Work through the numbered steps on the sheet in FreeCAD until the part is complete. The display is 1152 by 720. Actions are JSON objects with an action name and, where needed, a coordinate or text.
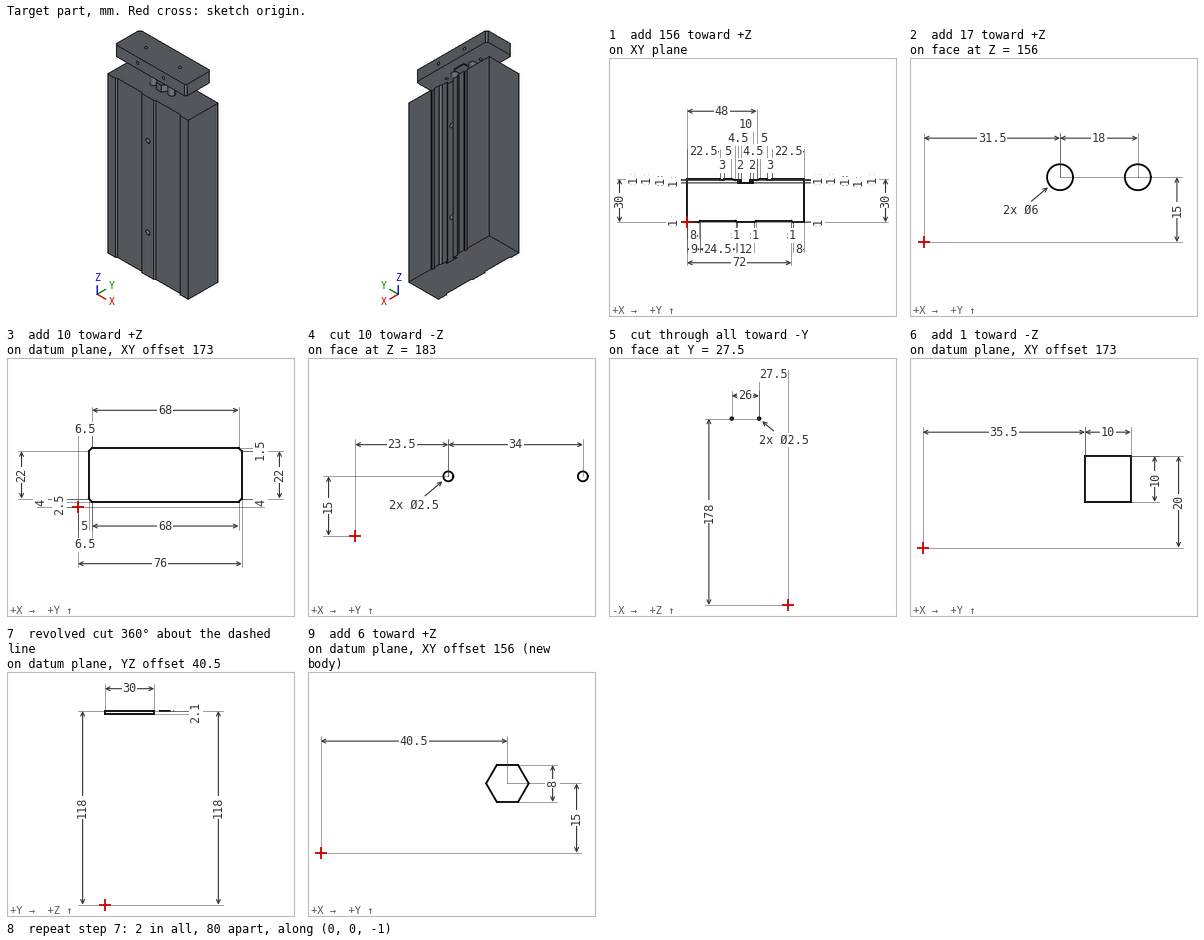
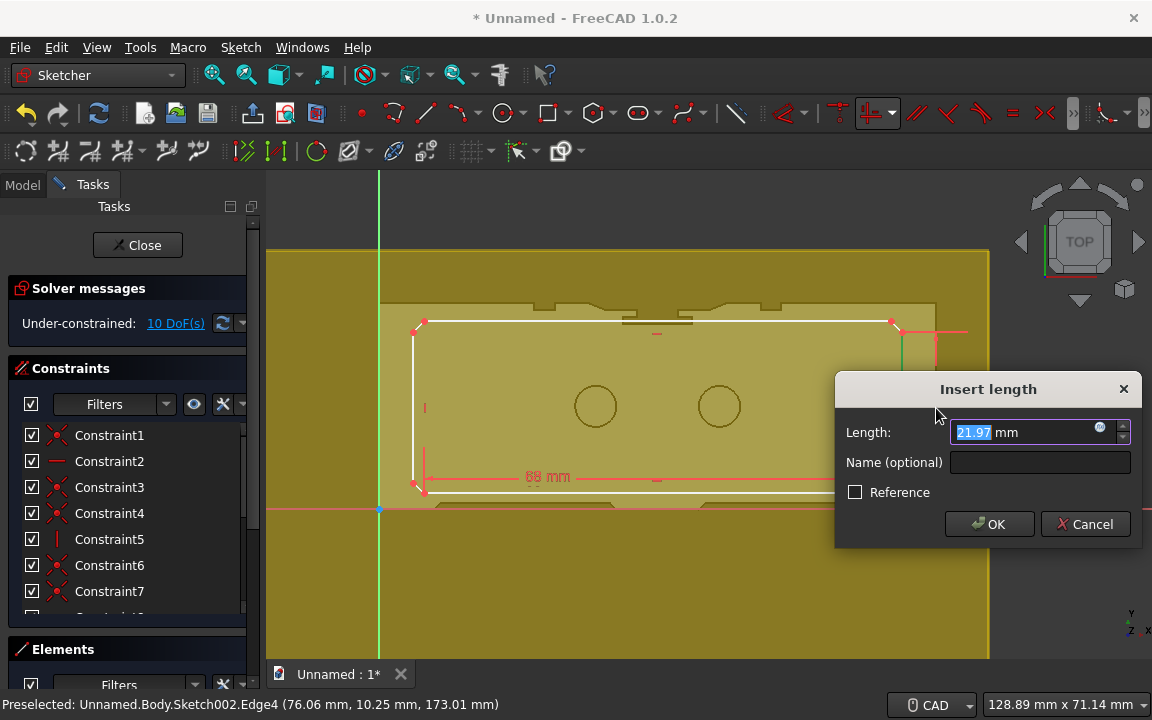
{"action": "type", "text": "22"}
{"action": "key", "text": "Return"}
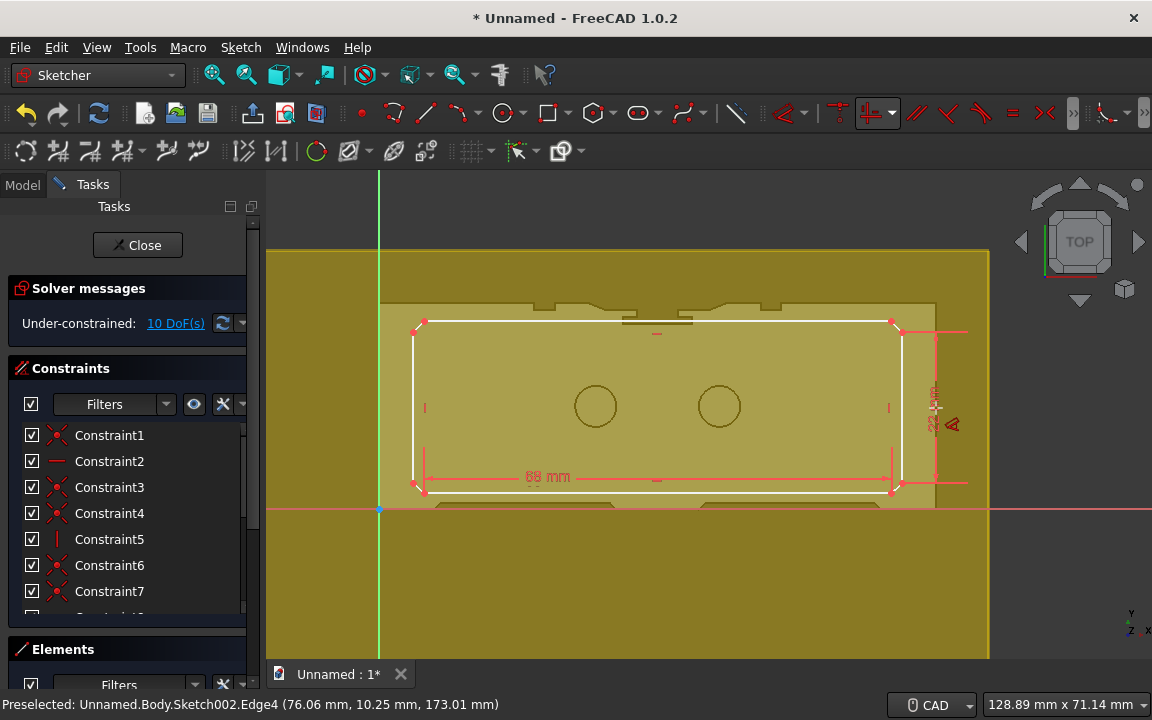
{"action": "left_click", "coordinate": [751, 321]}
{"action": "left_click", "coordinate": [658, 287]}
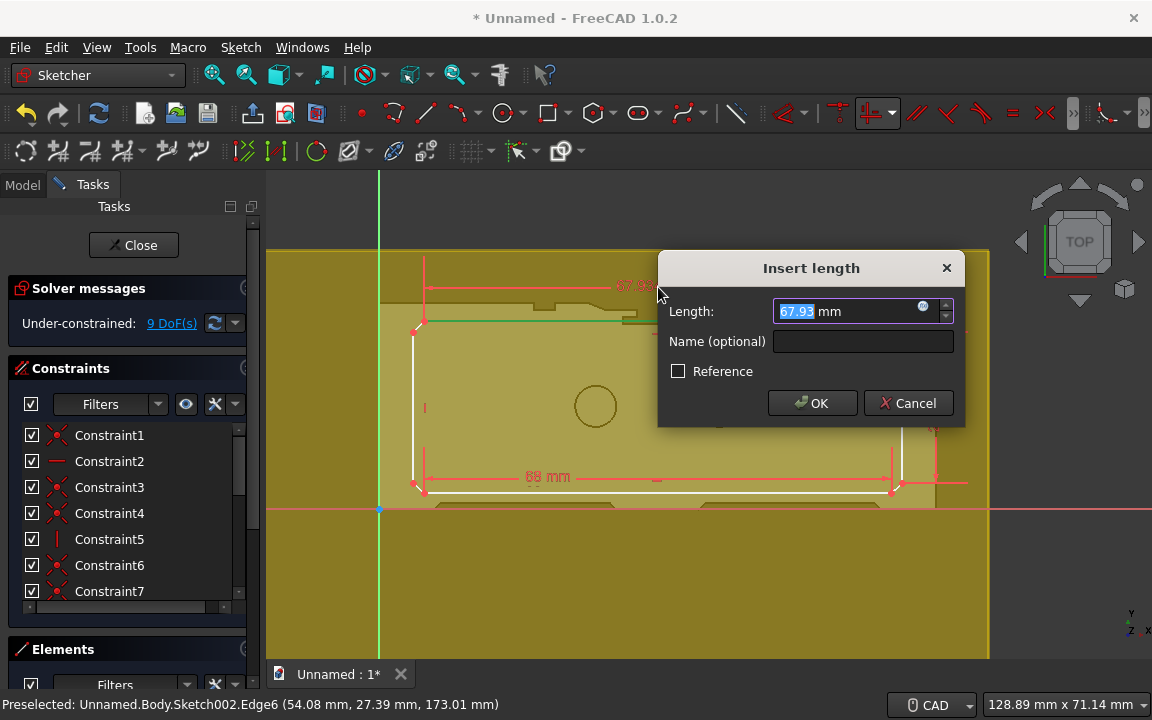
{"action": "type", "text": "68"}
{"action": "key", "text": "Return"}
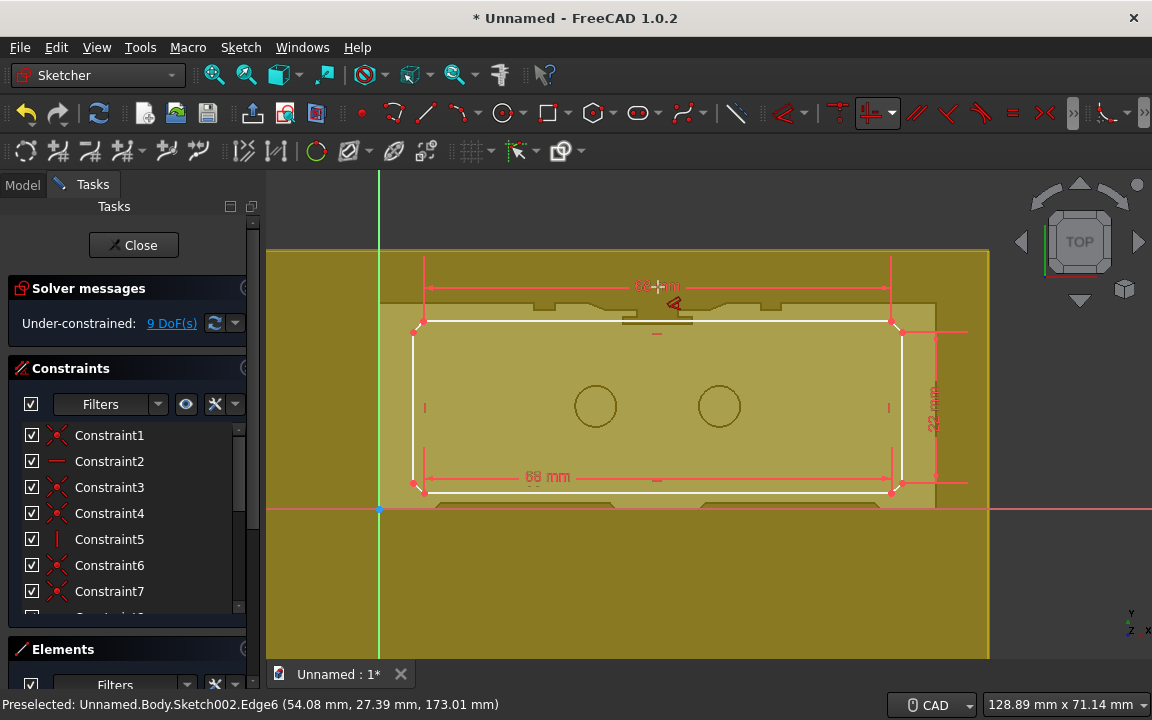
{"action": "left_click", "coordinate": [413, 378]}
{"action": "left_click", "coordinate": [447, 408]}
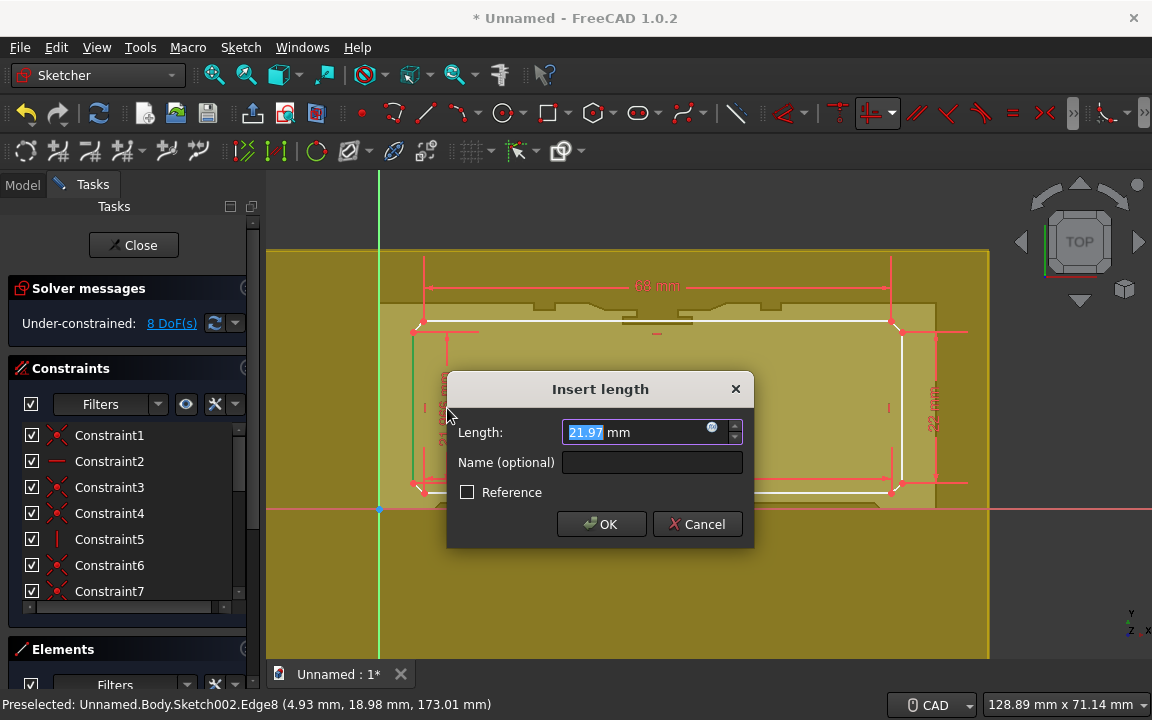
{"action": "type", "text": "22"}
{"action": "key", "text": "Return"}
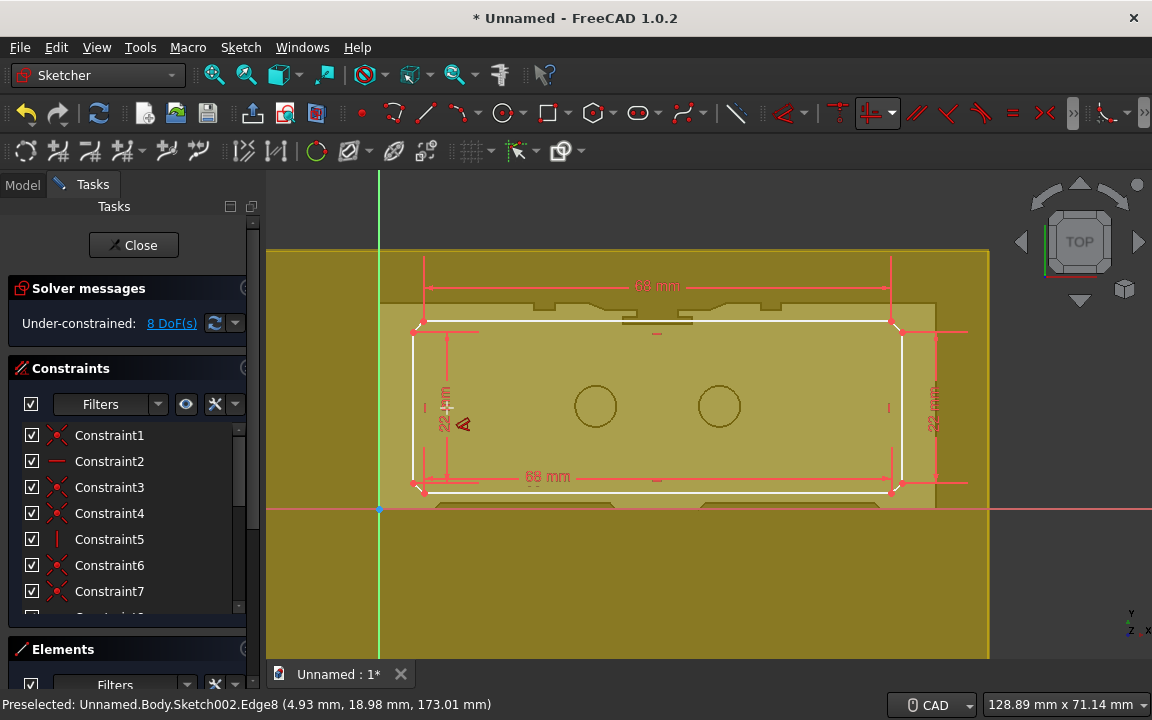
{"action": "left_click", "coordinate": [413, 483]}
{"action": "left_click", "coordinate": [396, 543]}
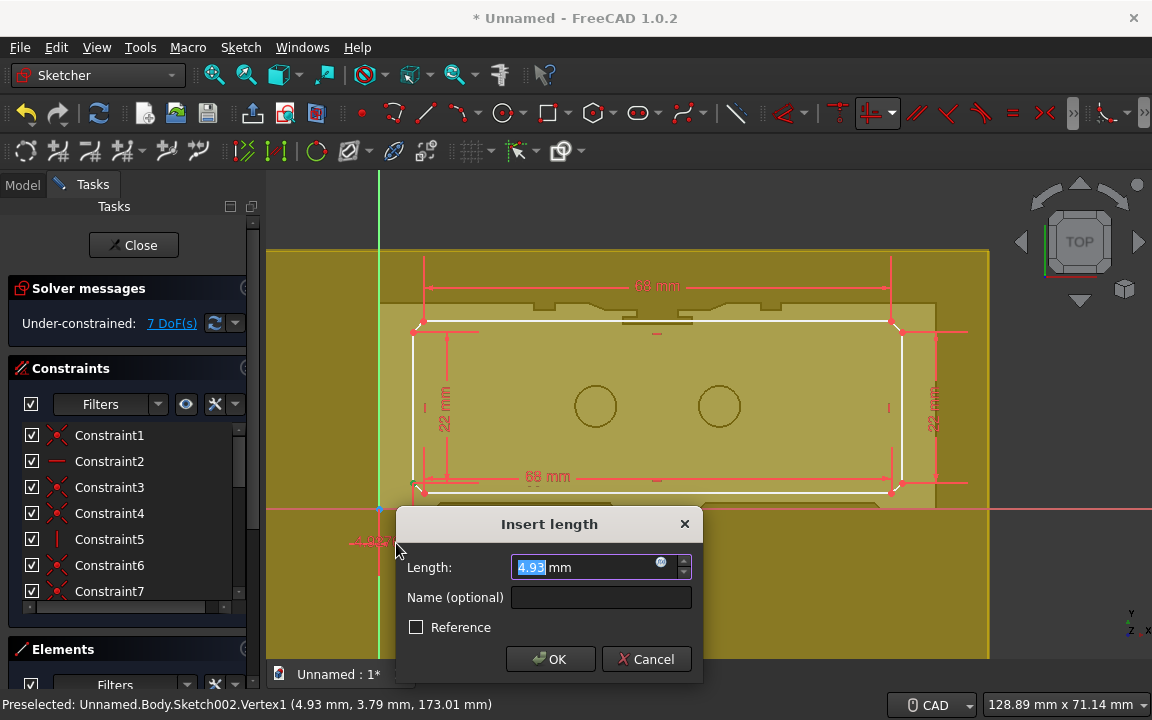
{"action": "type", "text": "5"}
{"action": "key", "text": "Return"}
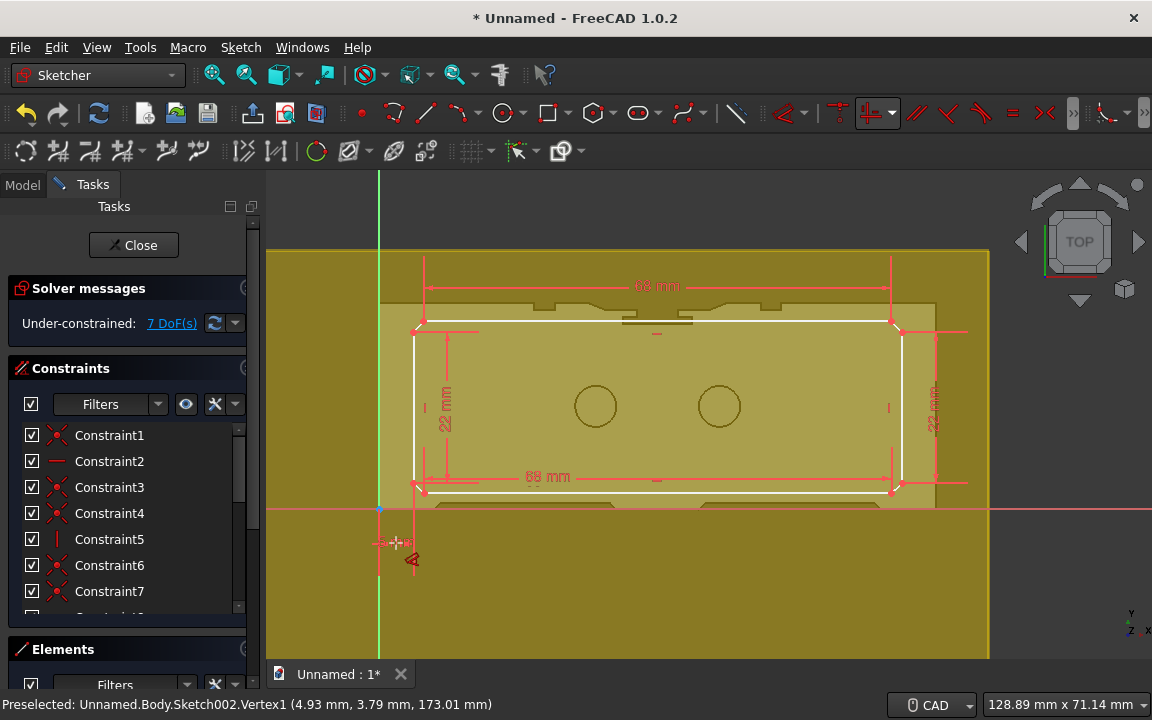
{"action": "scroll", "coordinate": [414, 483], "scroll_direction": "up", "scroll_amount": 2}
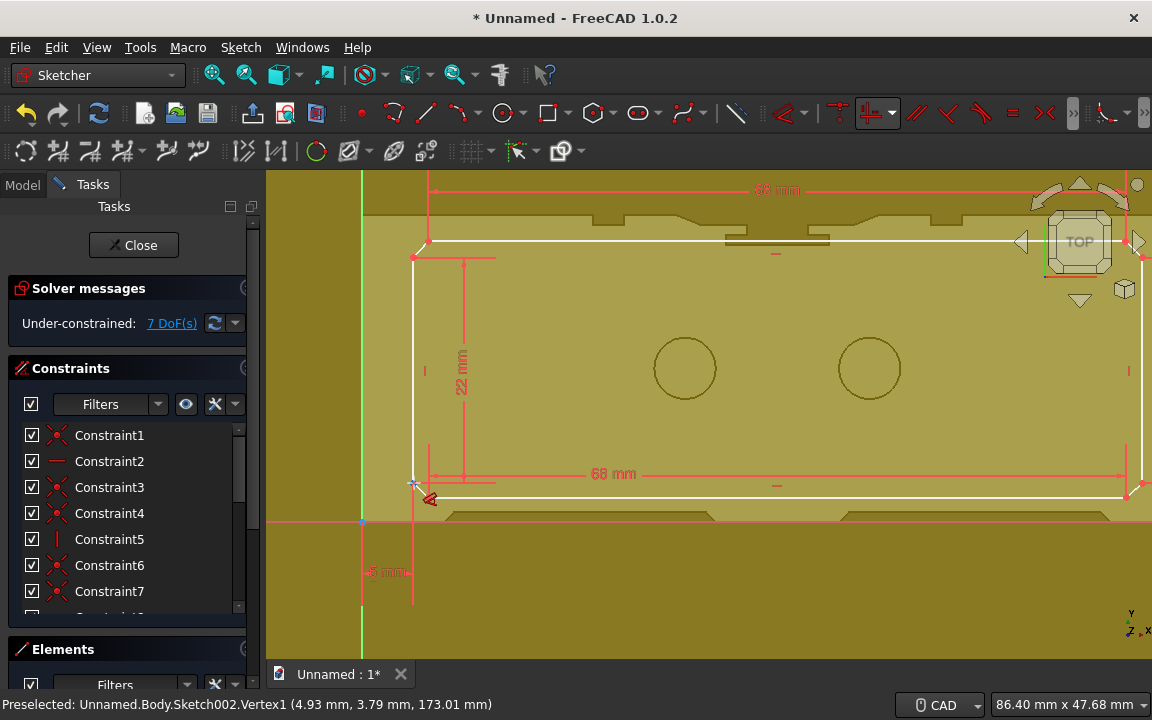
{"action": "left_click", "coordinate": [413, 483]}
{"action": "left_click", "coordinate": [328, 503]}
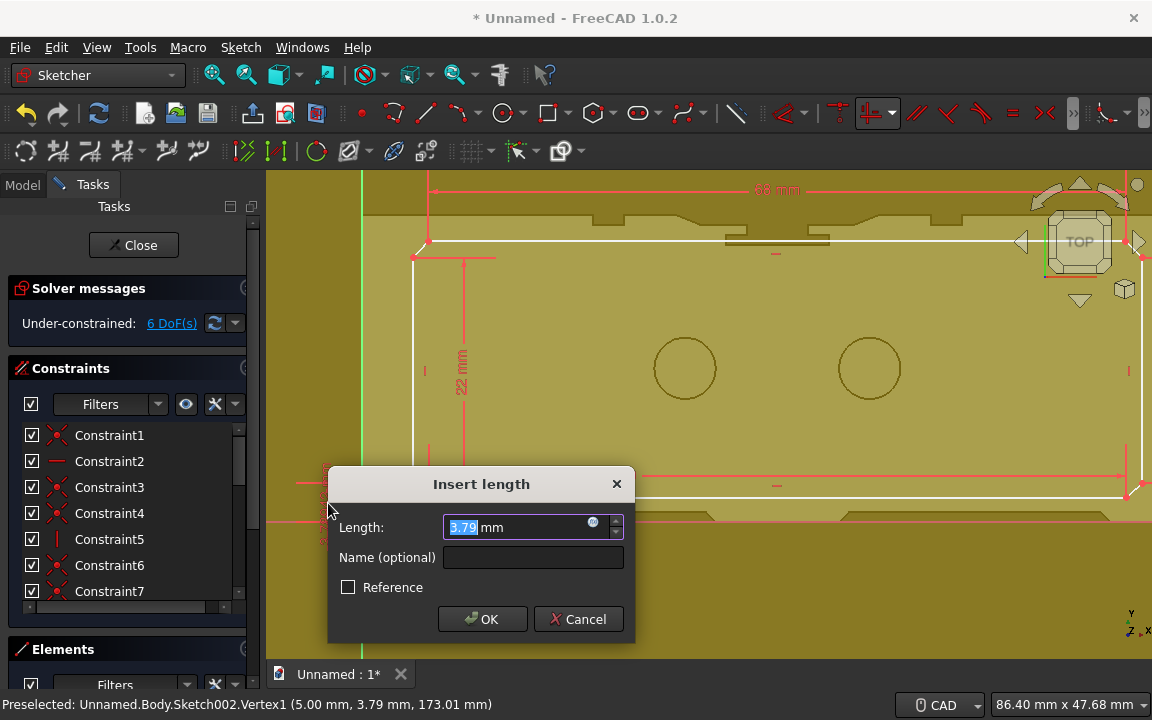
{"action": "type", "text": "4"}
{"action": "key", "text": "Return"}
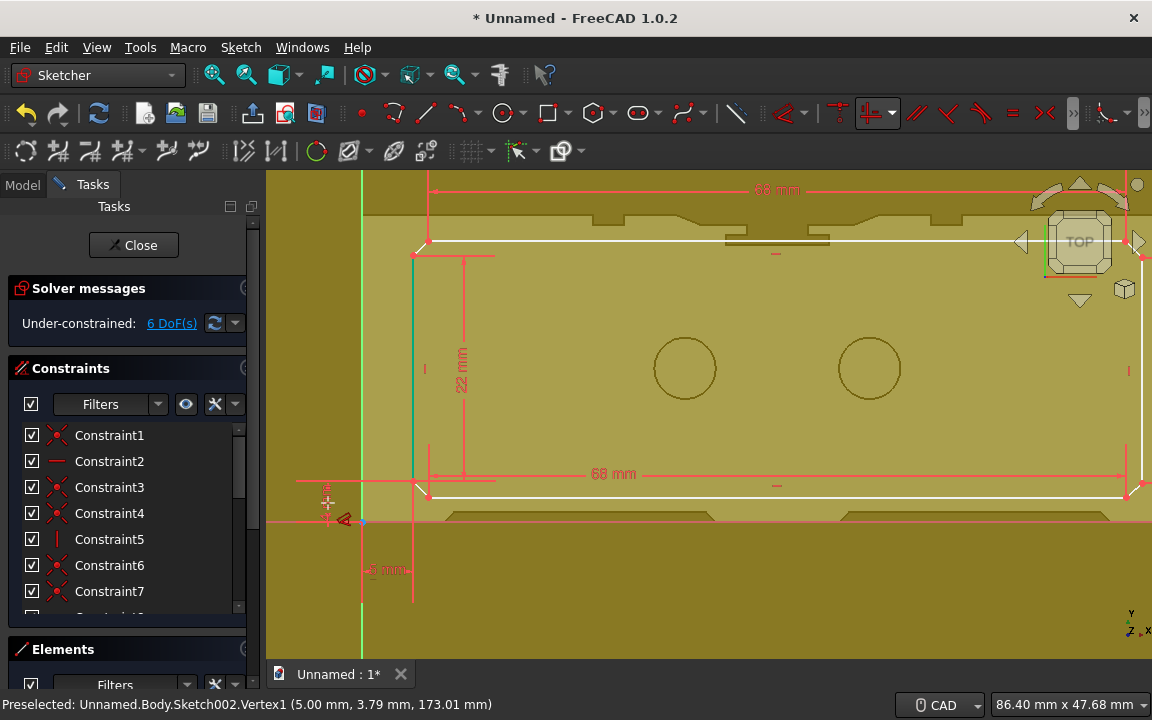
{"action": "scroll", "coordinate": [414, 482], "scroll_direction": "down", "scroll_amount": 2}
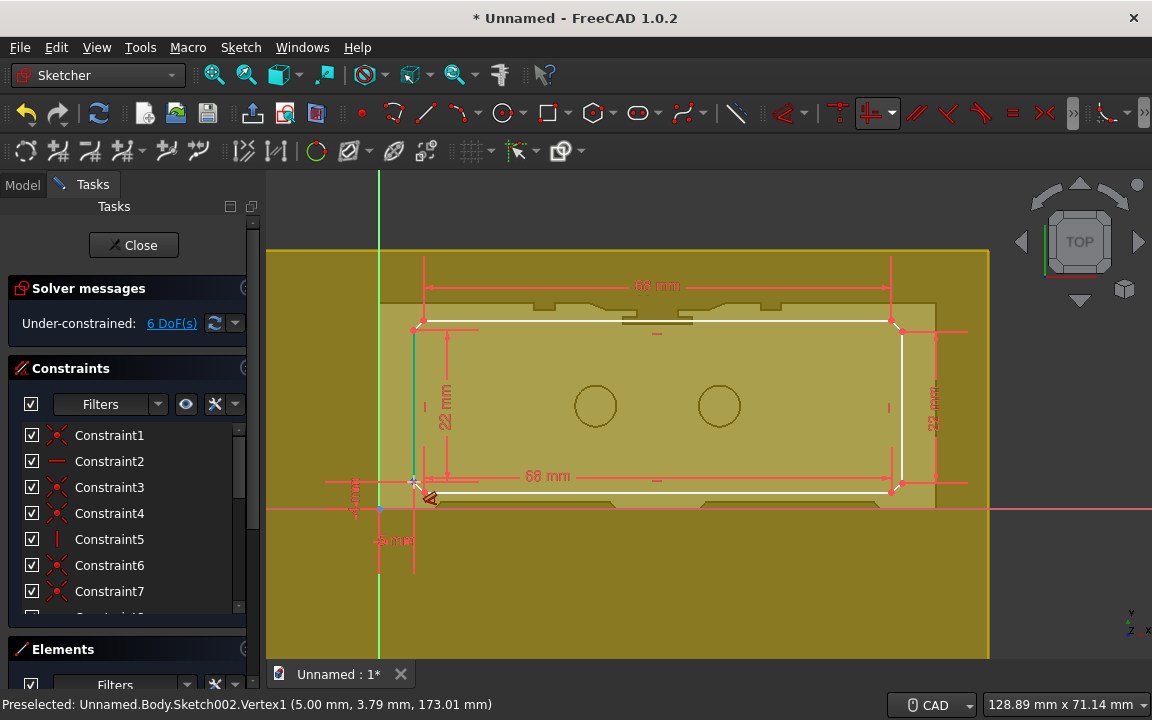
{"action": "scroll", "coordinate": [902, 483], "scroll_direction": "up", "scroll_amount": 2}